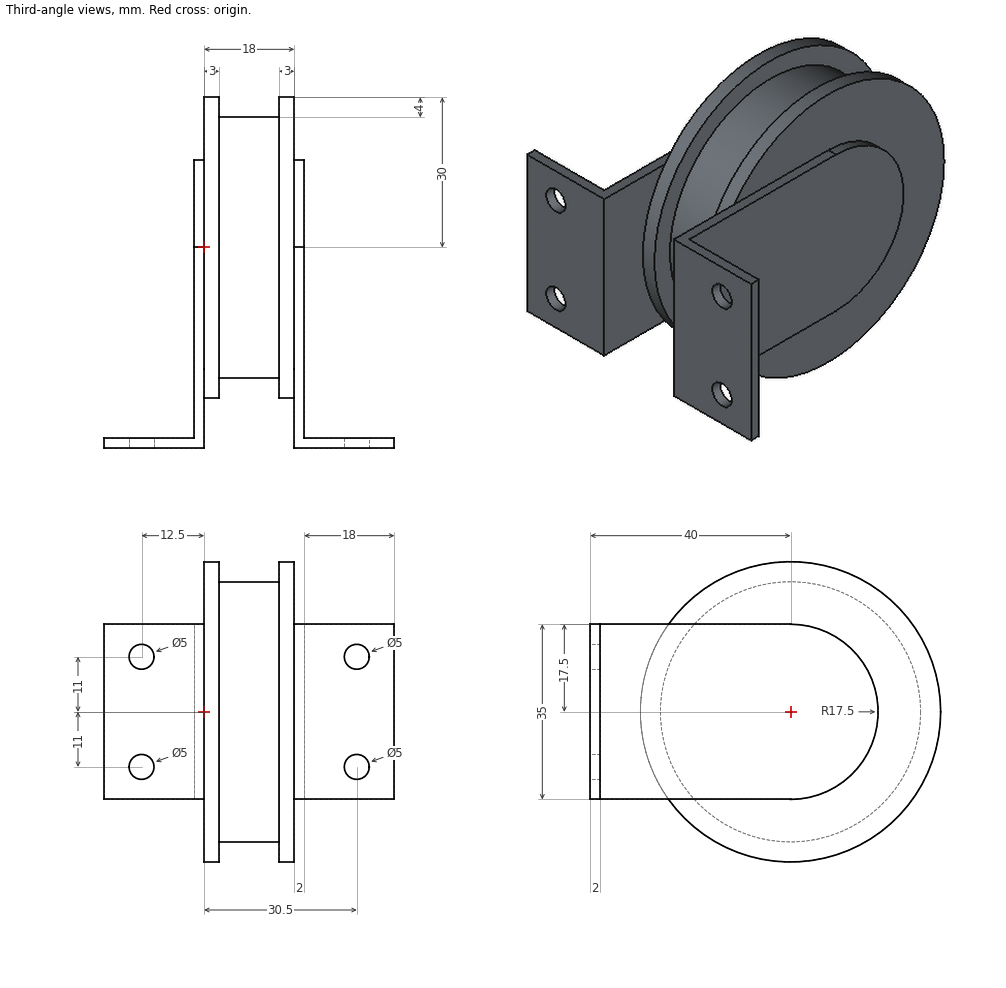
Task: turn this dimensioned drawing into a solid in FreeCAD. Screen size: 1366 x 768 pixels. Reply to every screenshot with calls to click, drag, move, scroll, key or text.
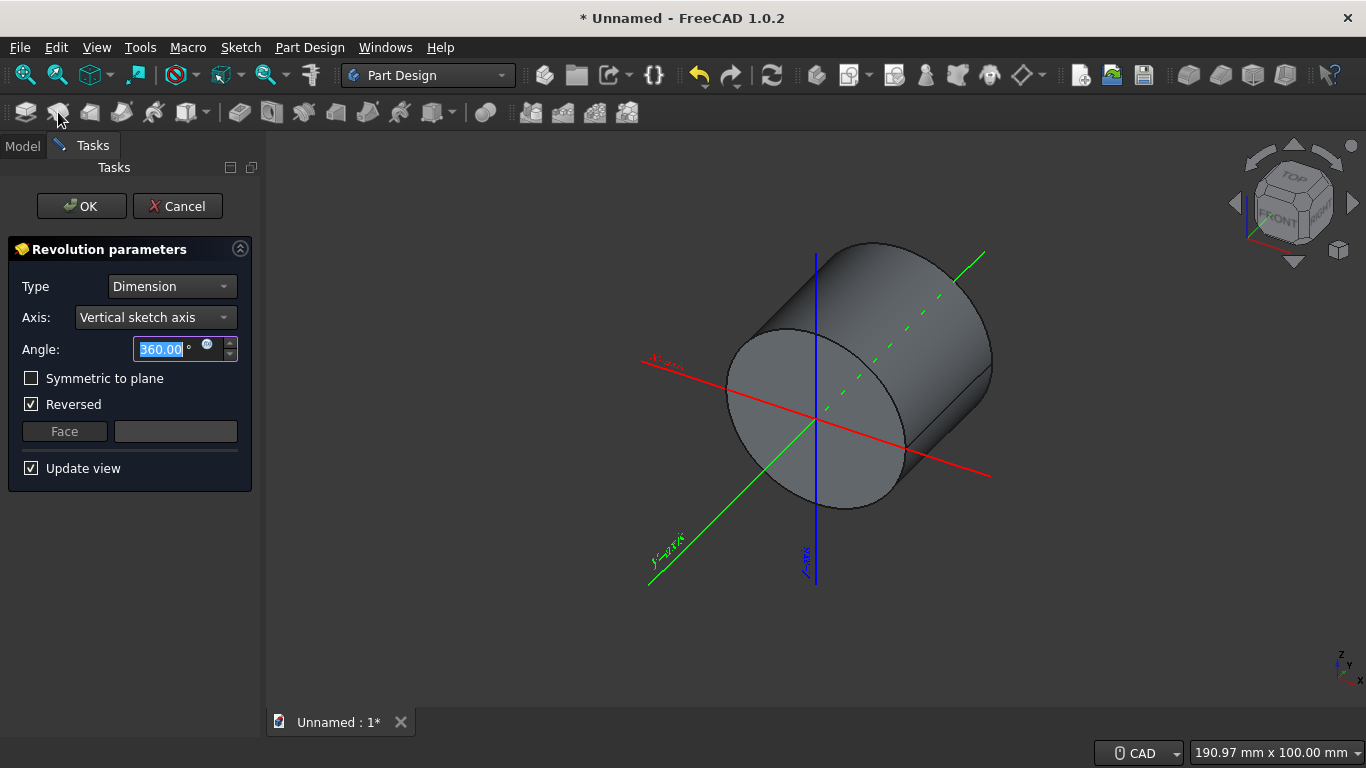
click(156, 318)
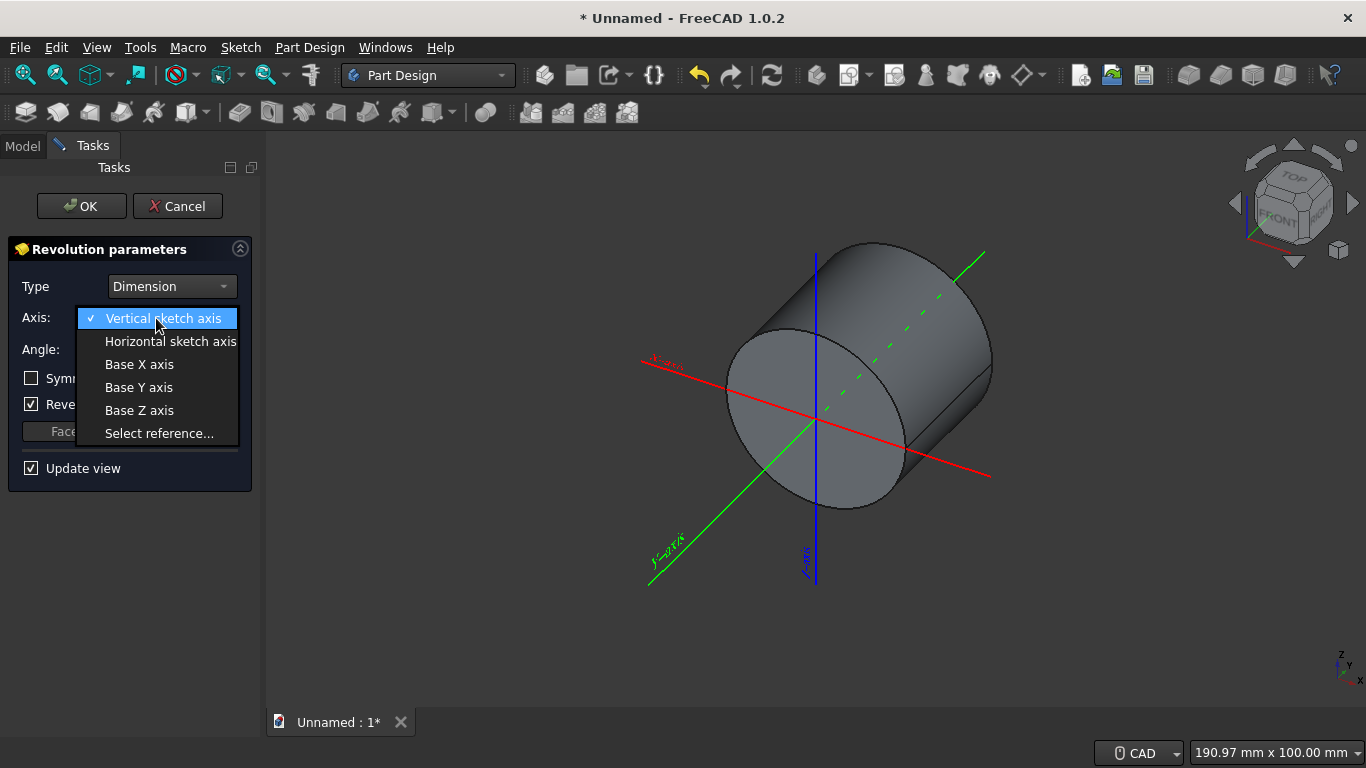
click(156, 342)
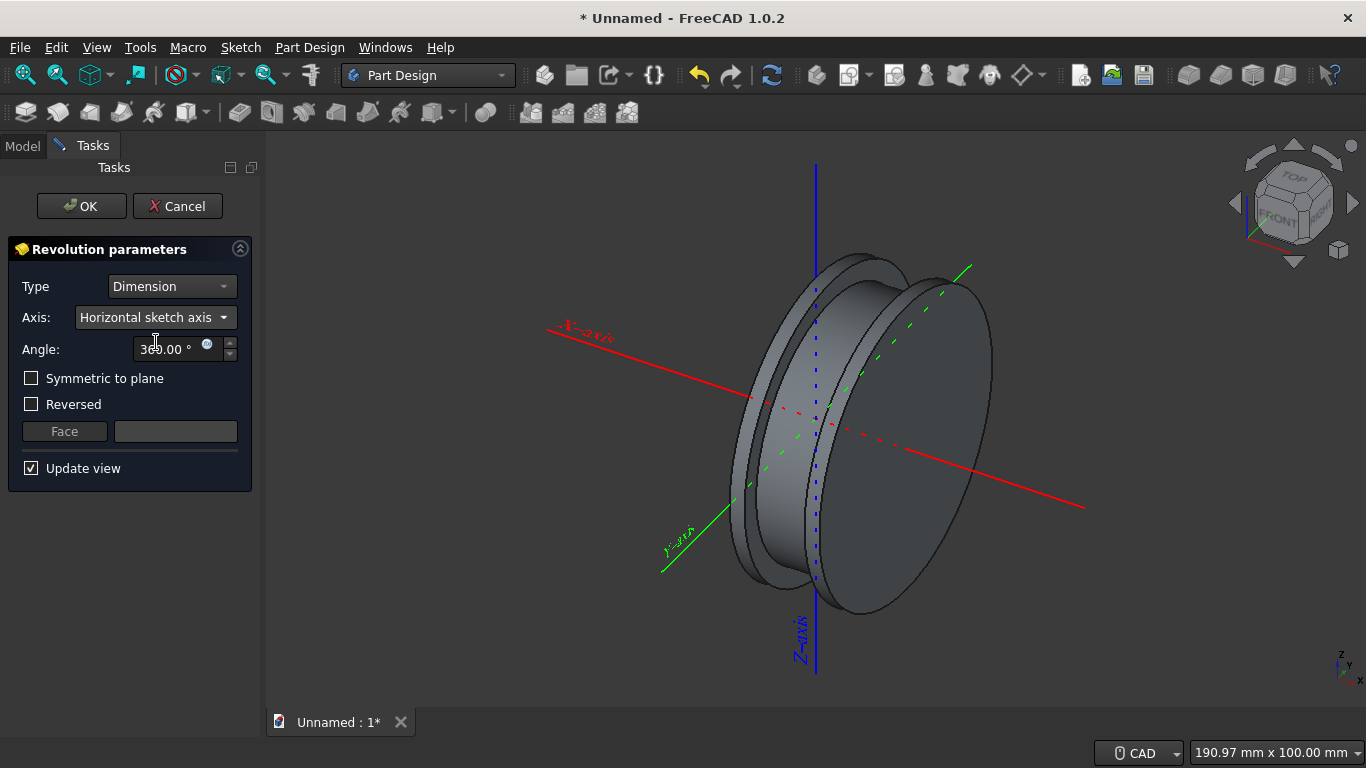
click(82, 206)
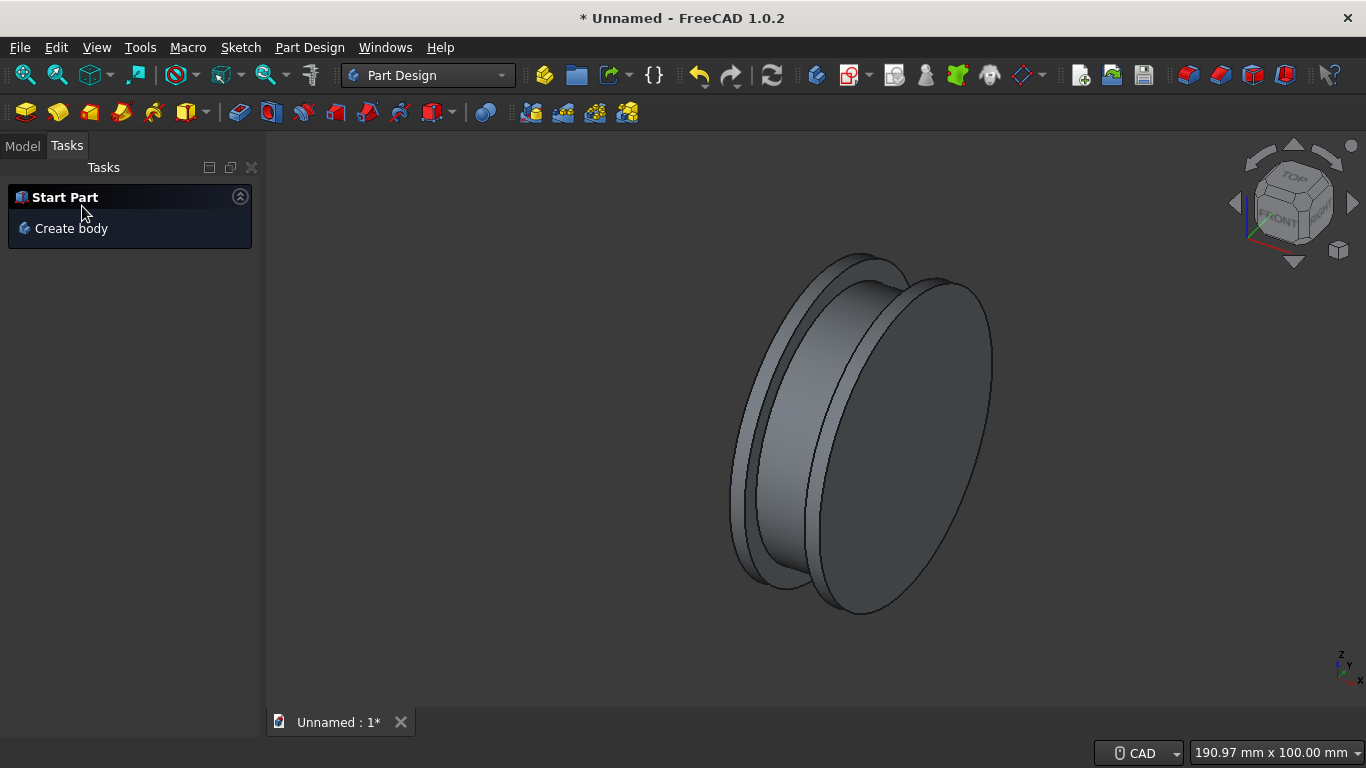
click(906, 448)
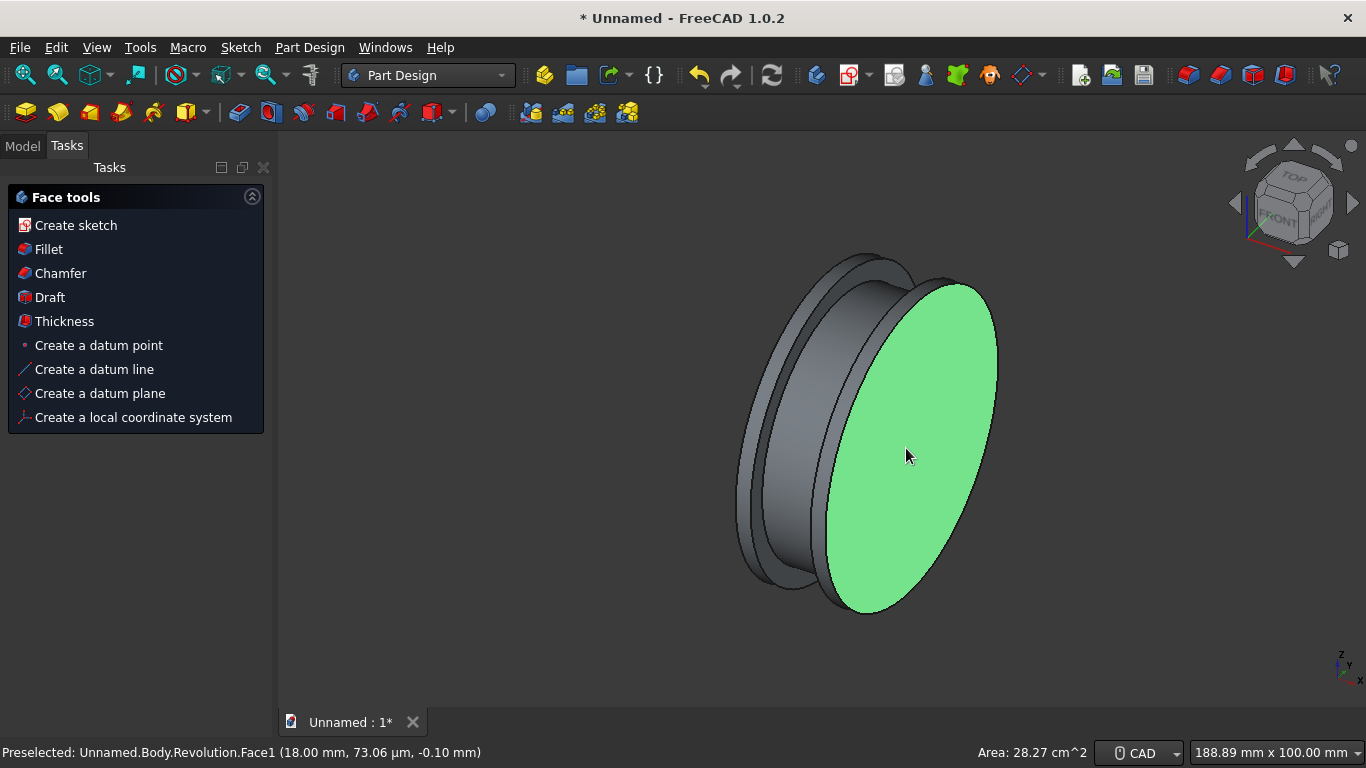
click(850, 76)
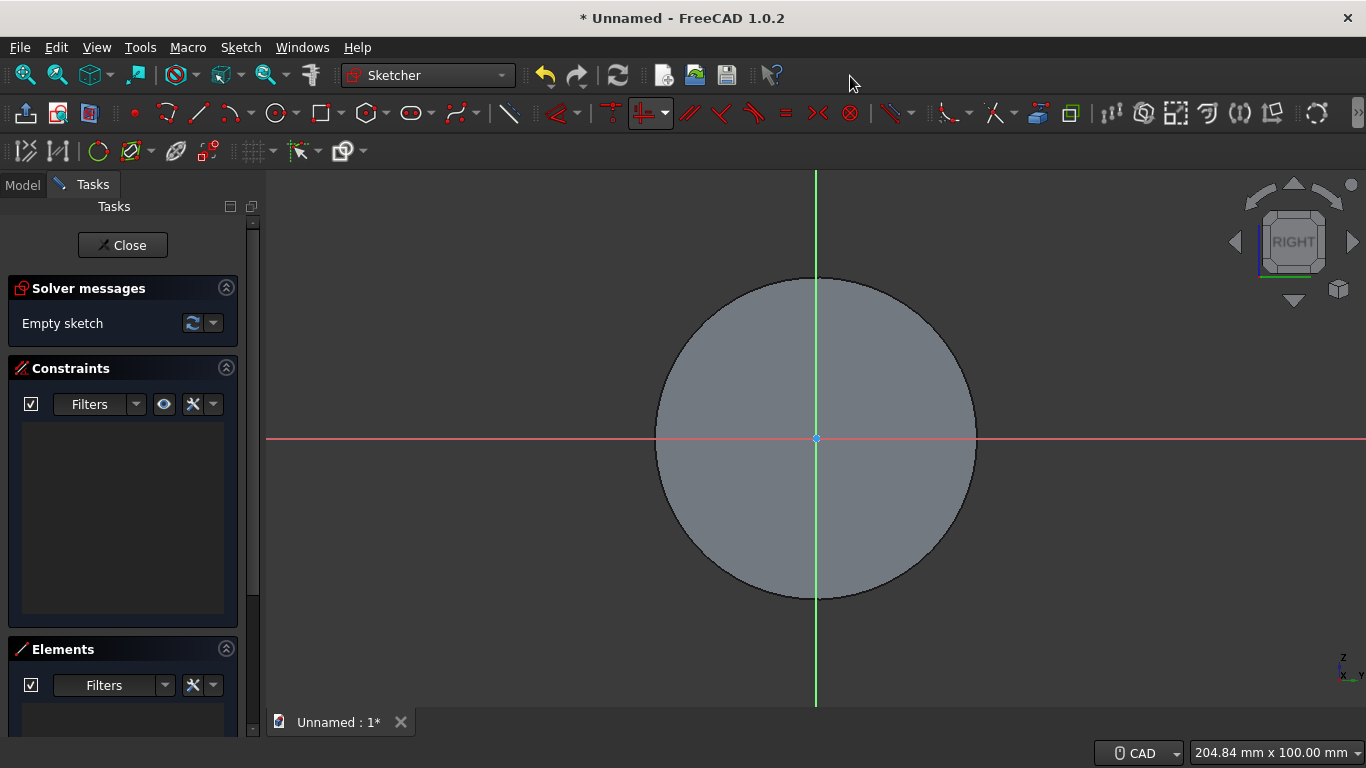
scroll(765, 438, up, 3)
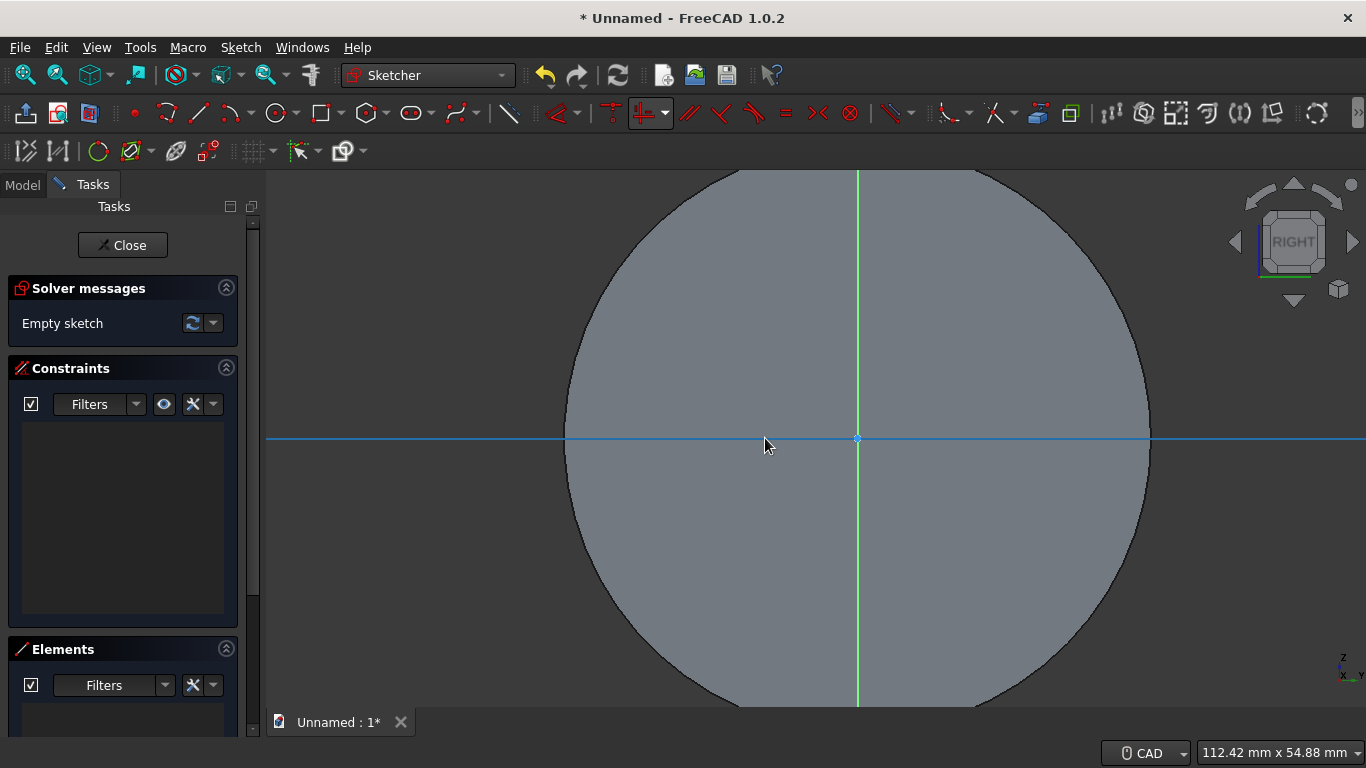
click(168, 114)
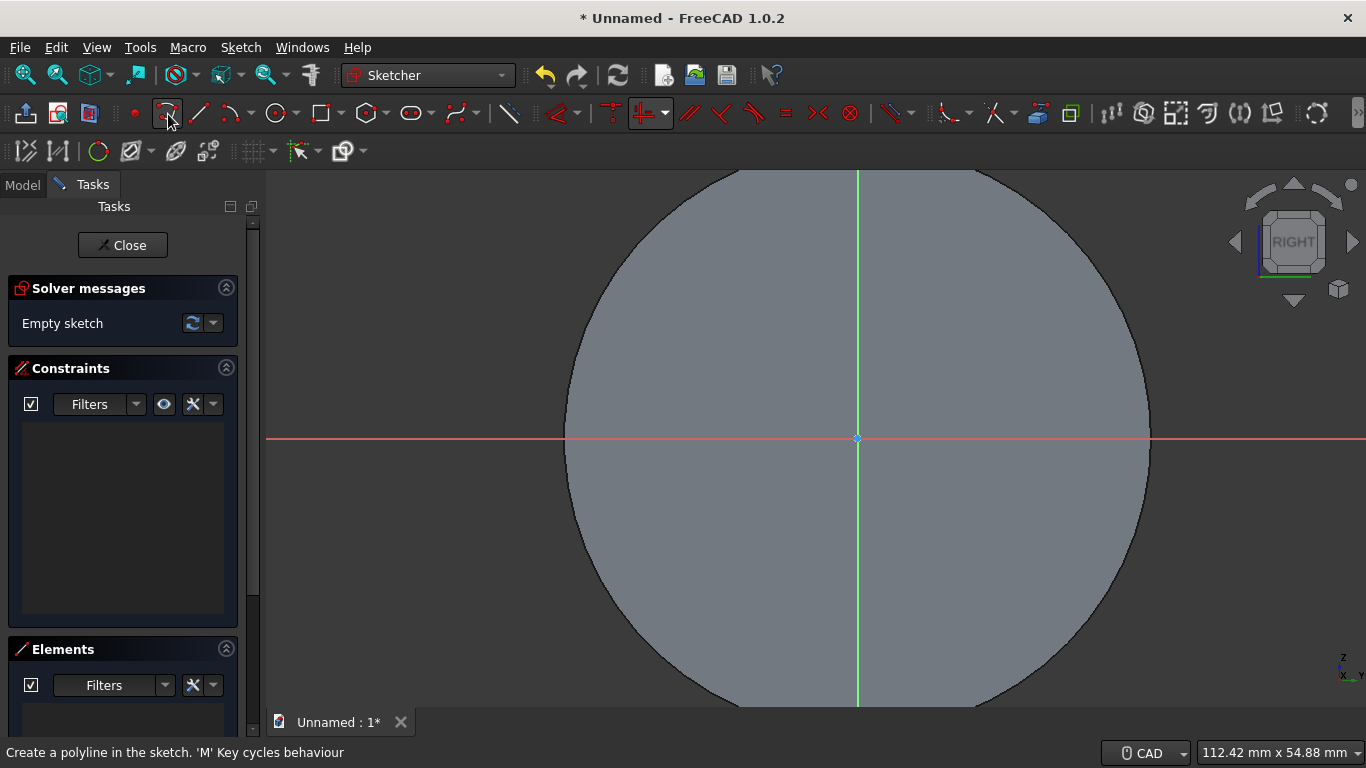
click(858, 267)
click(466, 267)
click(466, 610)
click(858, 610)
right_click(858, 610)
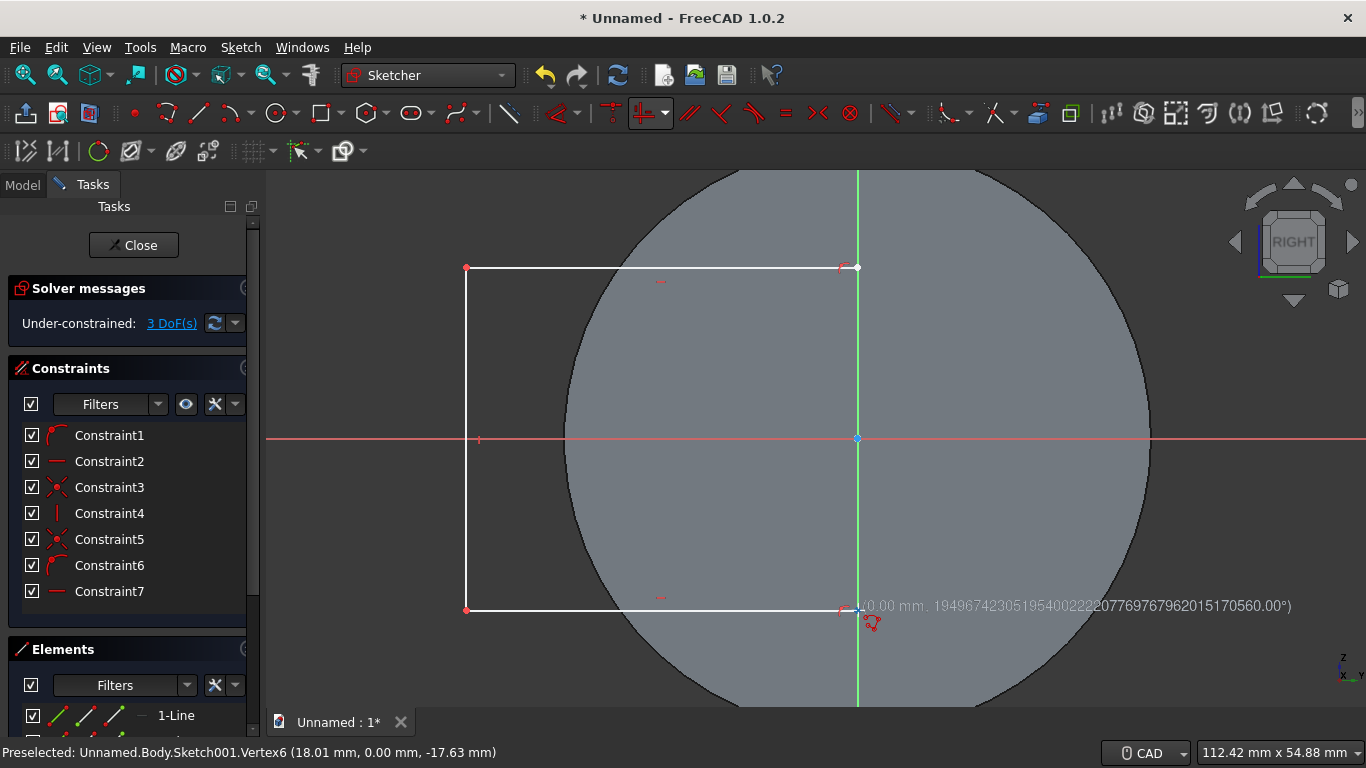
key(g)
key(3)
key(a)